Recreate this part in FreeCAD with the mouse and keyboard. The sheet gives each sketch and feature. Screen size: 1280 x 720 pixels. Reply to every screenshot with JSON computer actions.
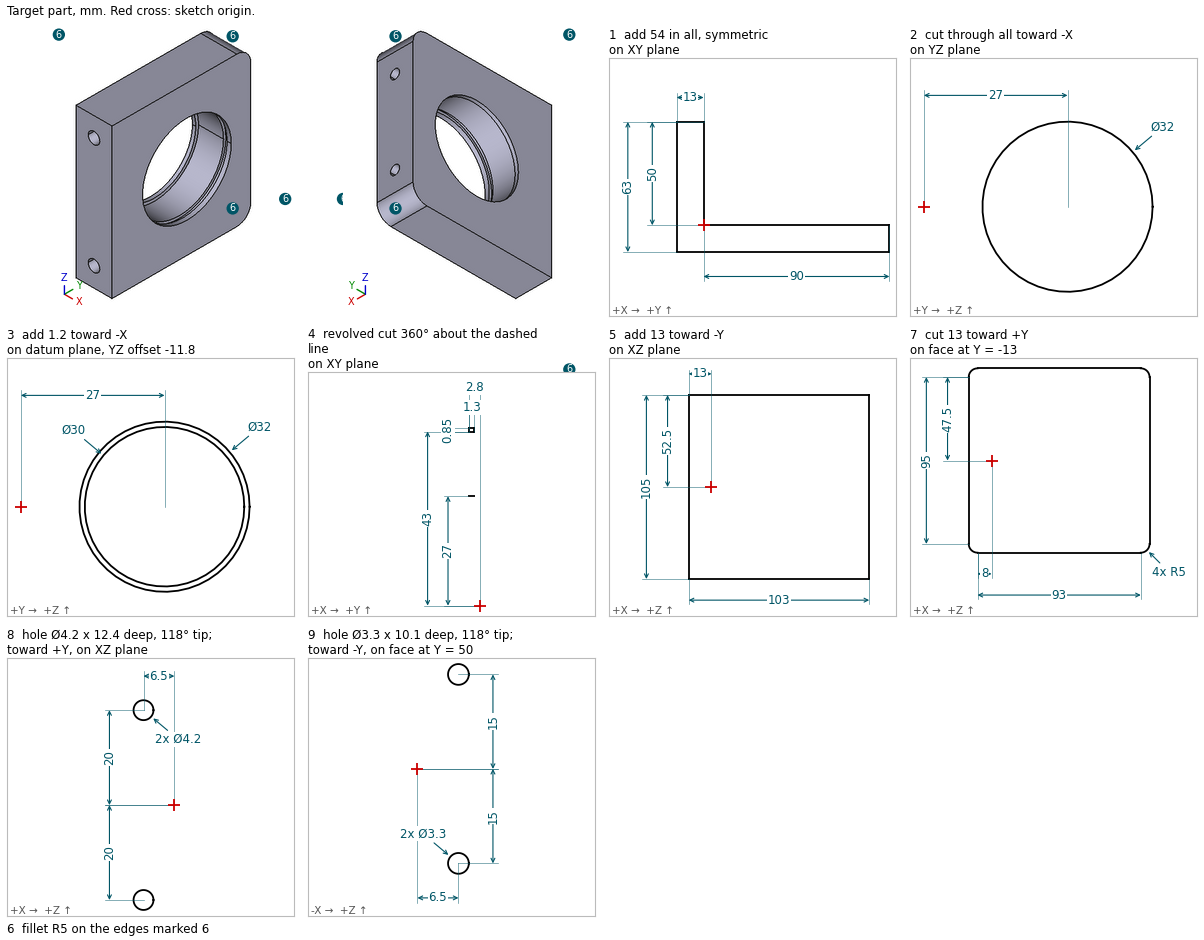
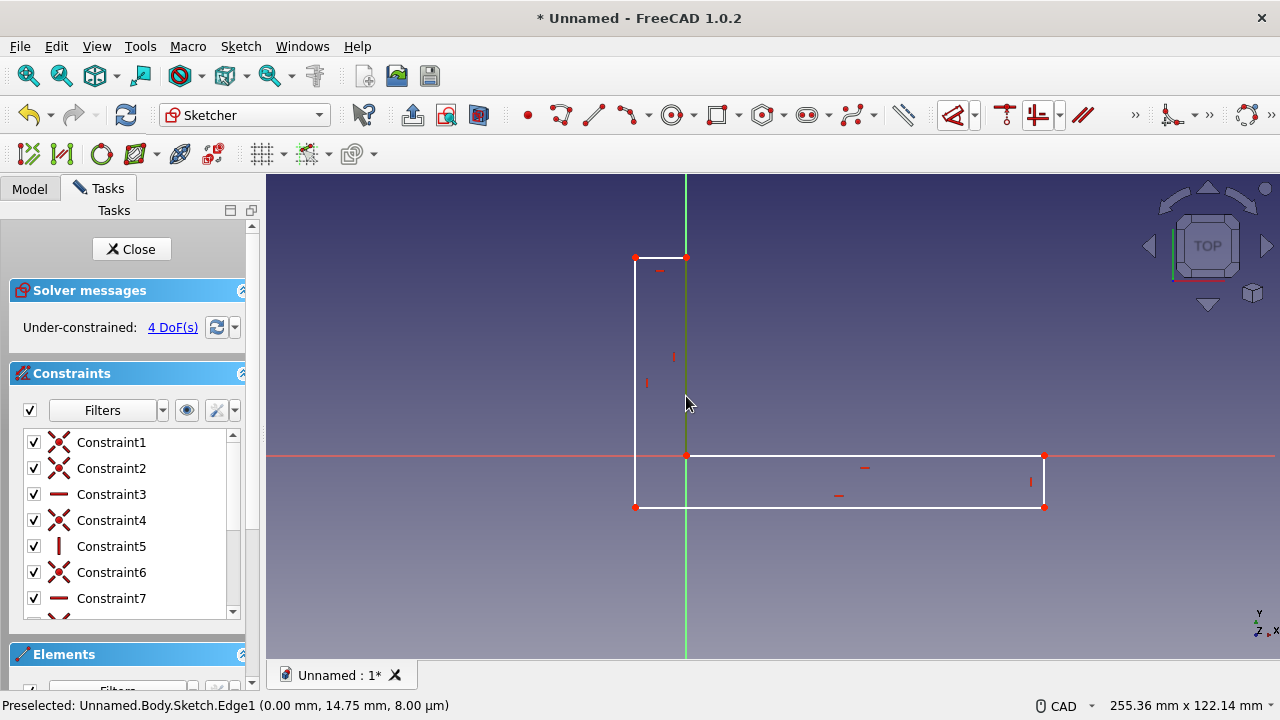
{"action": "left_click", "coordinate": [974, 116]}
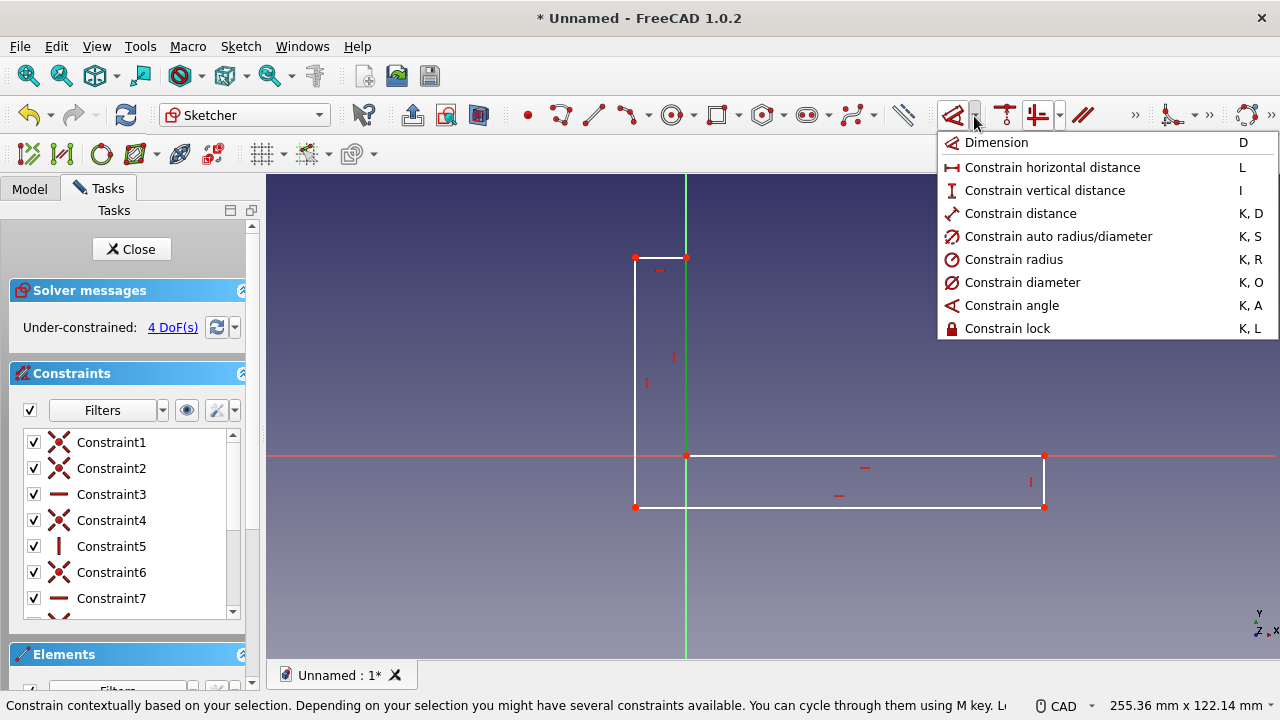
{"action": "left_click", "coordinate": [1108, 190]}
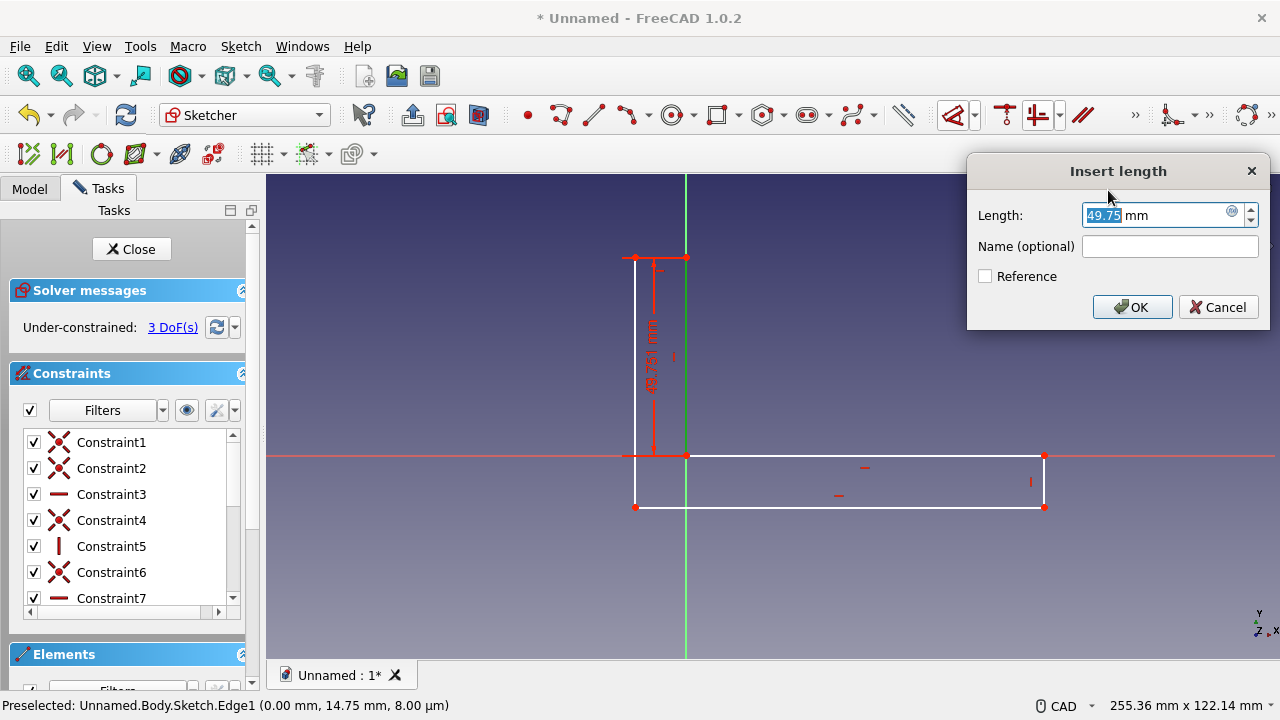
{"action": "type", "text": "50"}
{"action": "key", "text": "Return"}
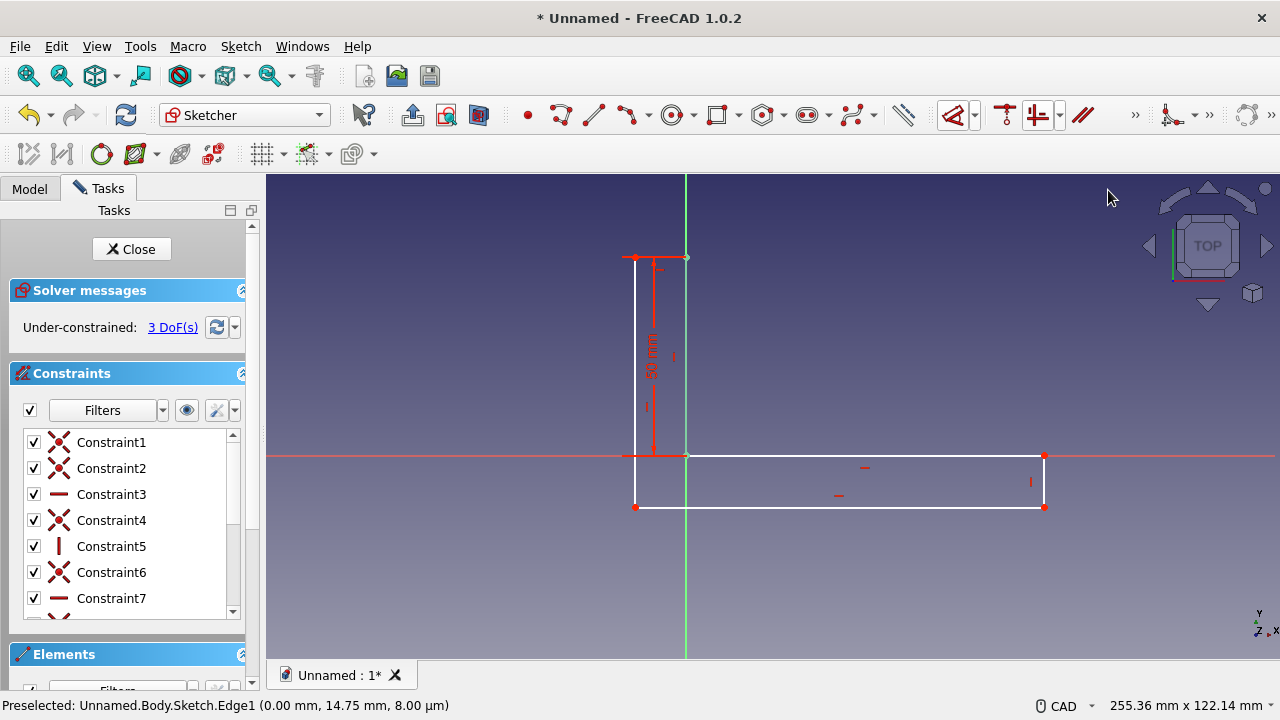
{"action": "left_click", "coordinate": [671, 257]}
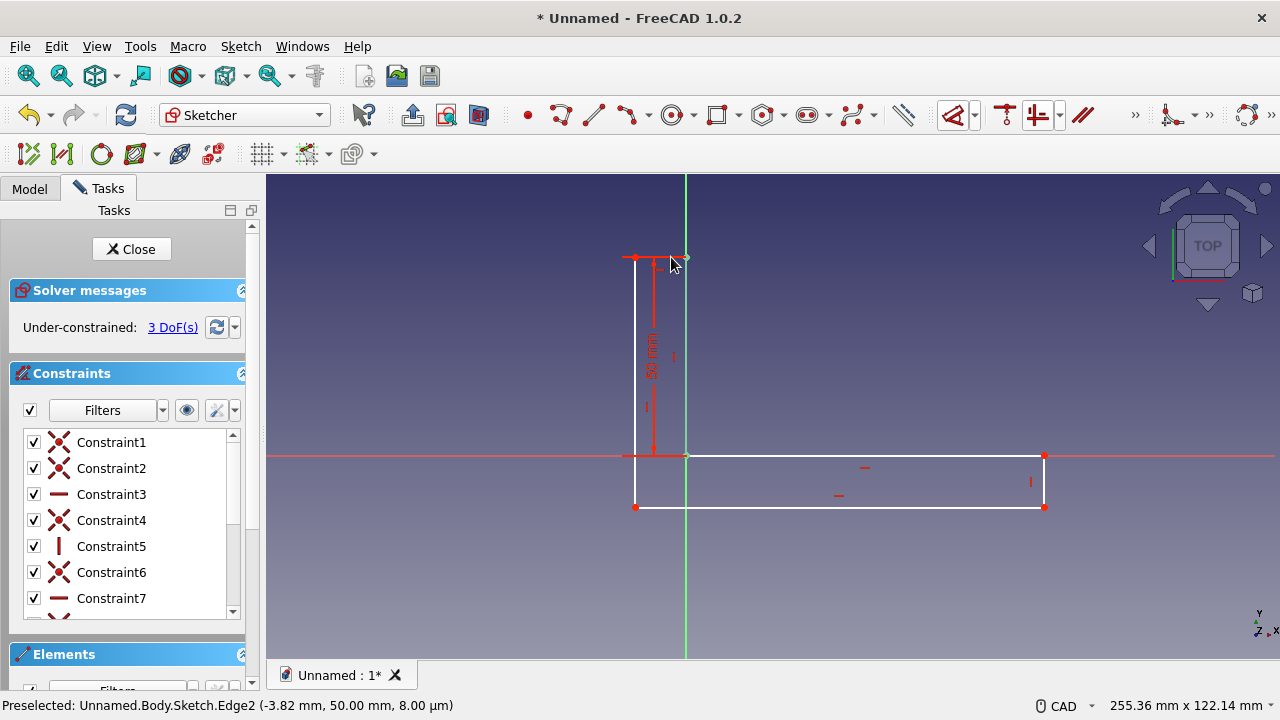
{"action": "left_click", "coordinate": [974, 116]}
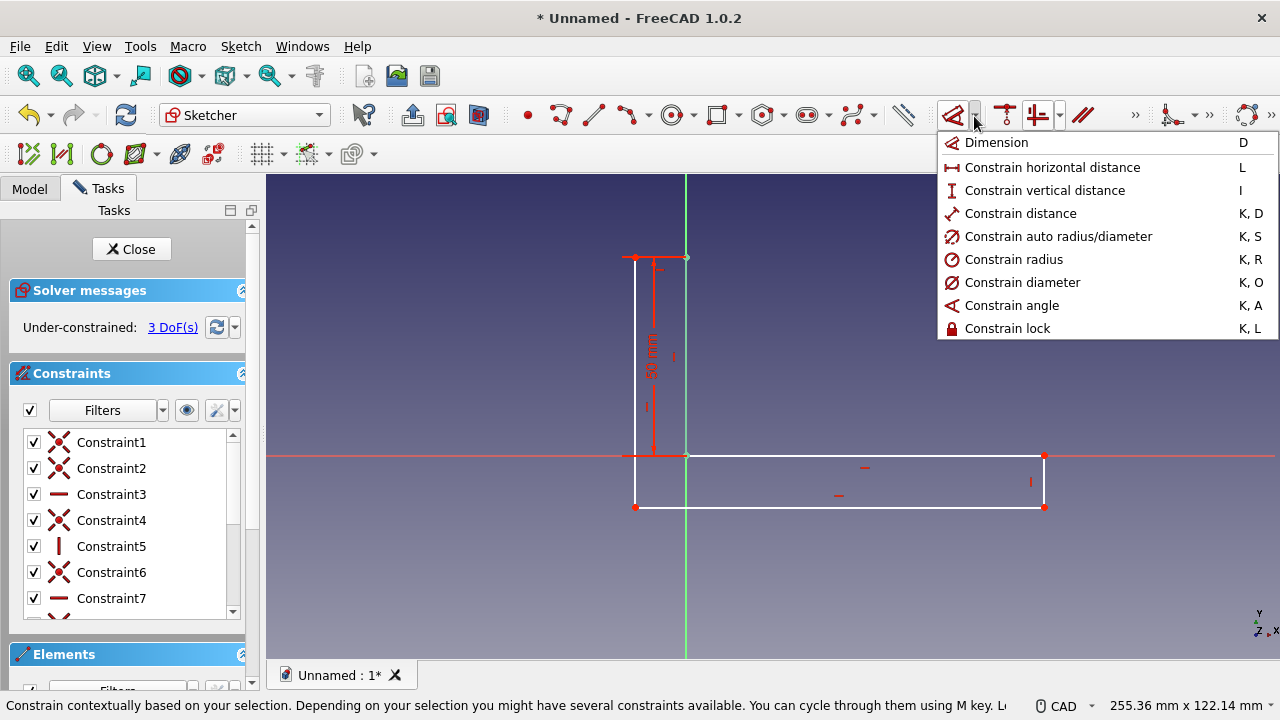
{"action": "left_click", "coordinate": [1108, 168]}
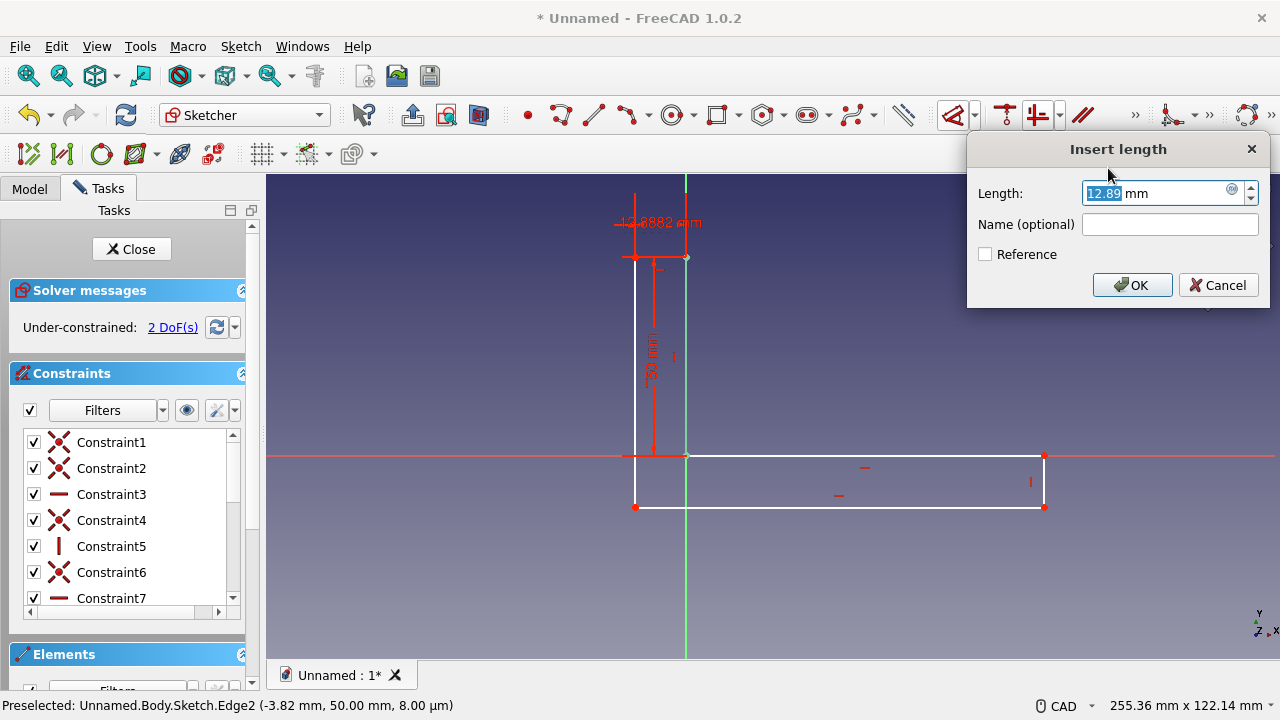
{"action": "type", "text": "13"}
{"action": "key", "text": "Return"}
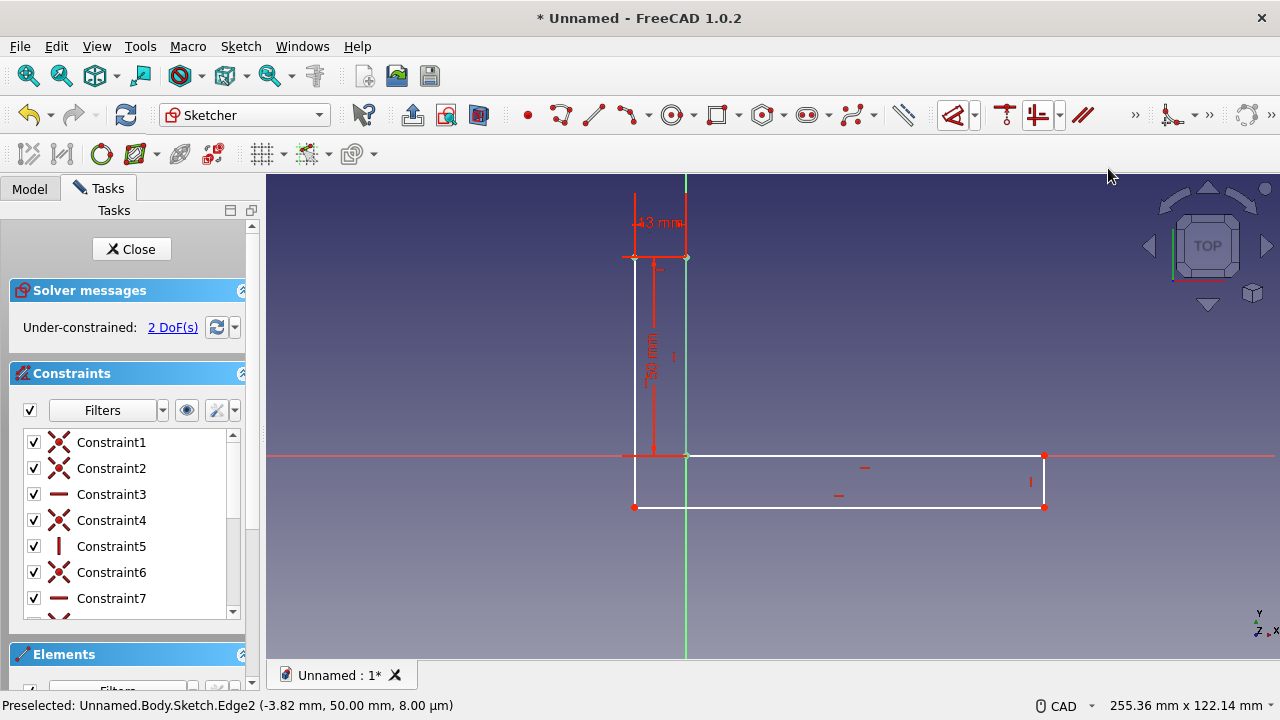
{"action": "left_click", "coordinate": [635, 332]}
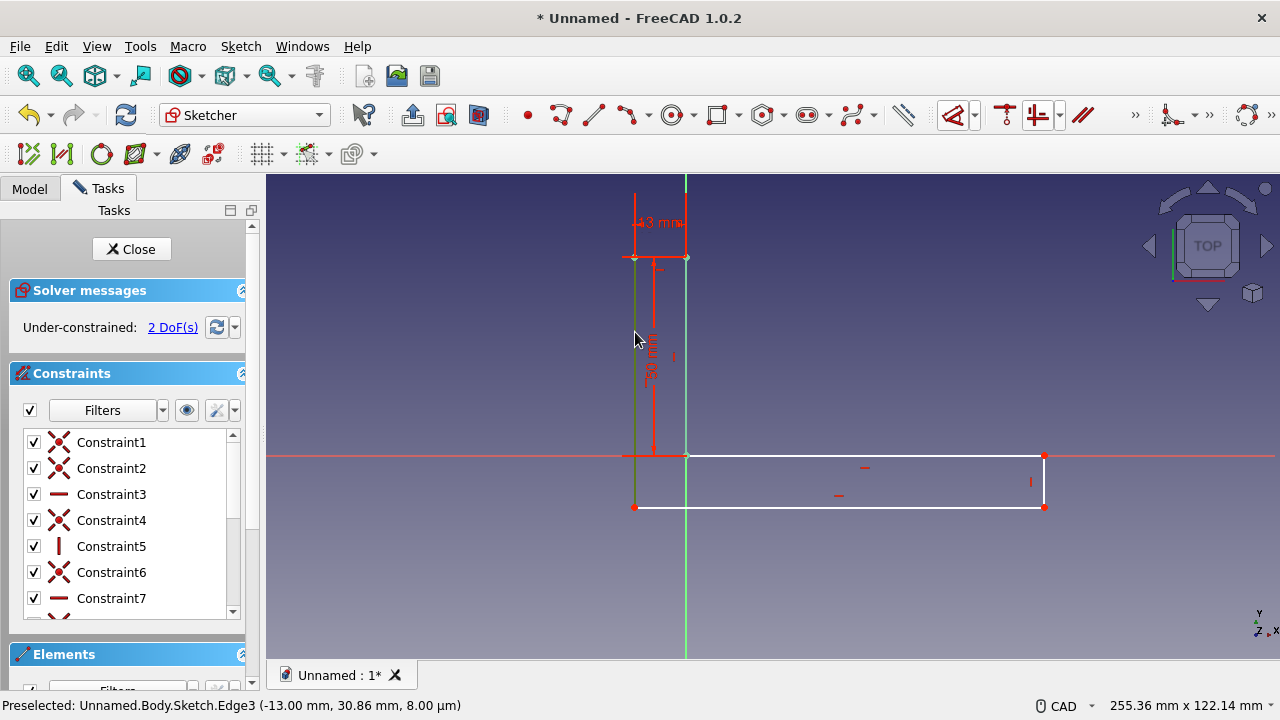
{"action": "key", "text": "i"}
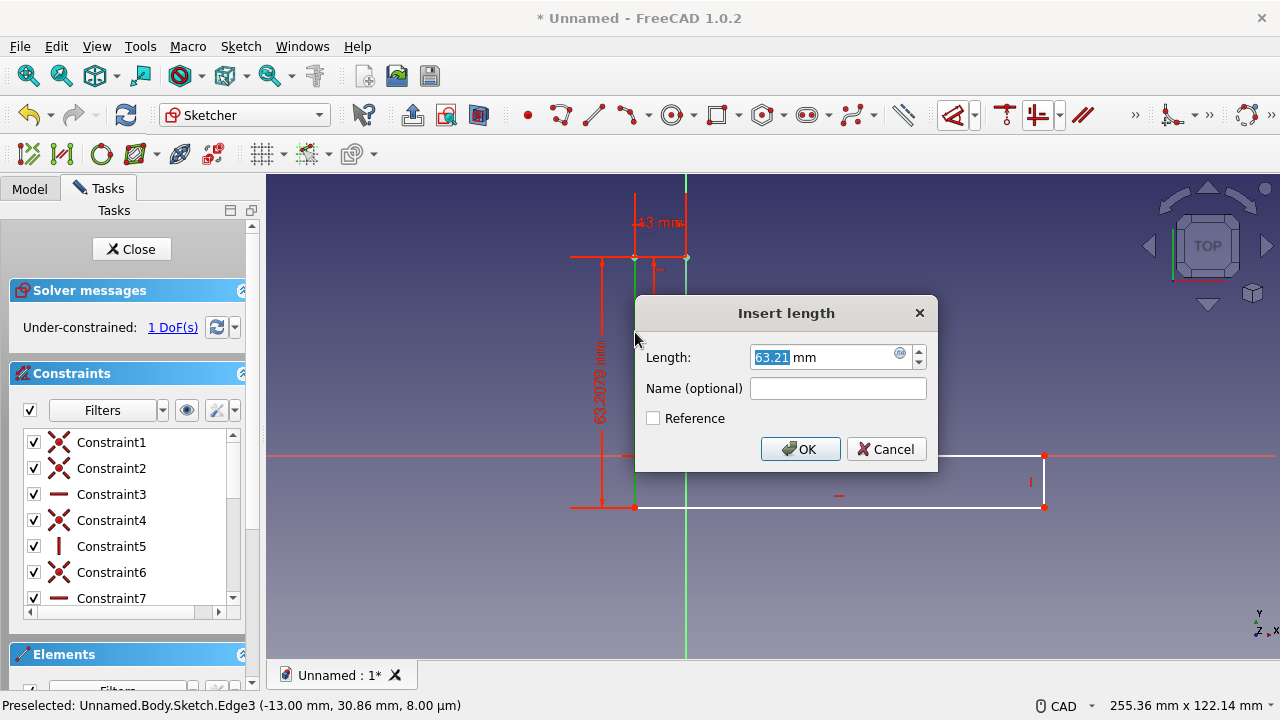
{"action": "type", "text": "63"}
{"action": "key", "text": "Return"}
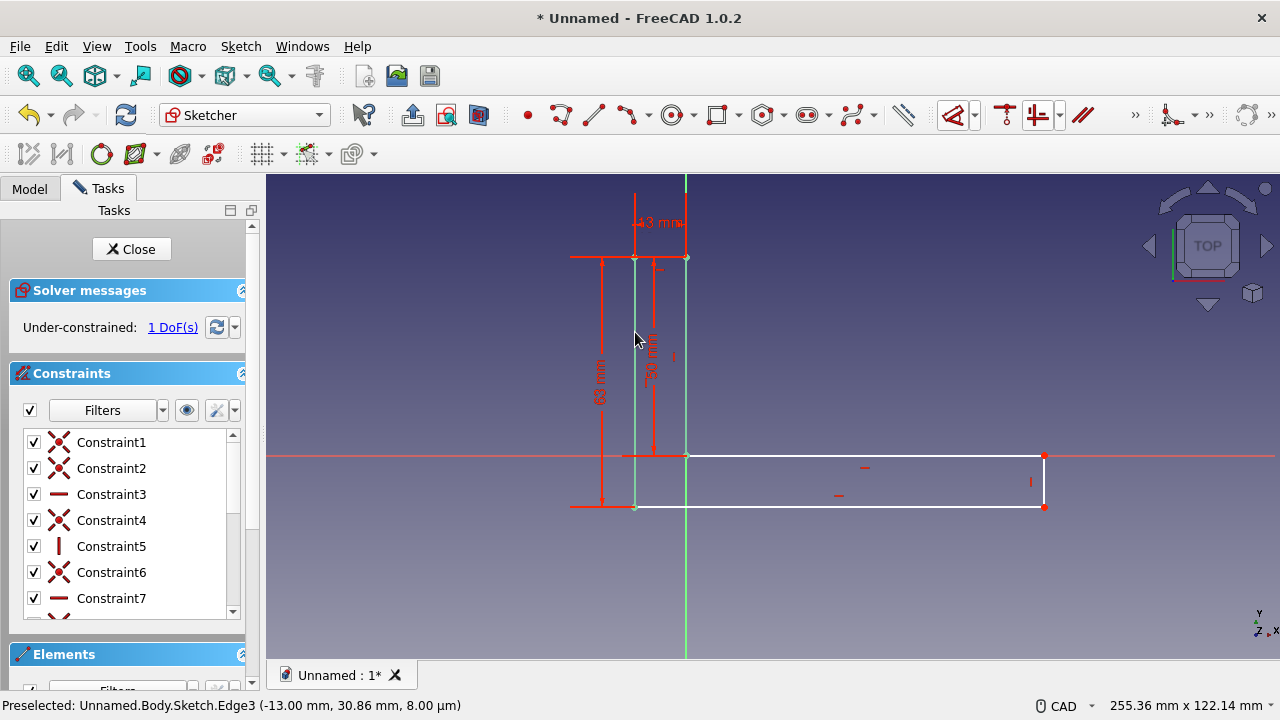
{"action": "left_click", "coordinate": [937, 456]}